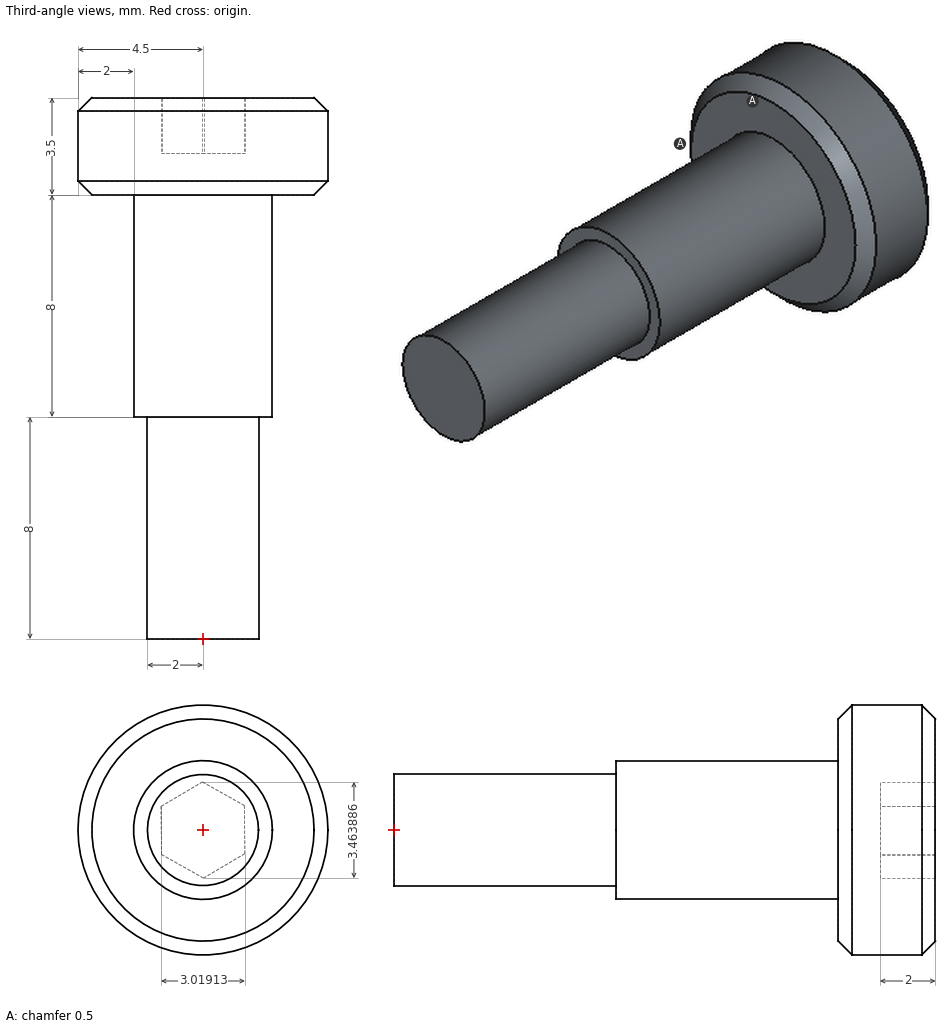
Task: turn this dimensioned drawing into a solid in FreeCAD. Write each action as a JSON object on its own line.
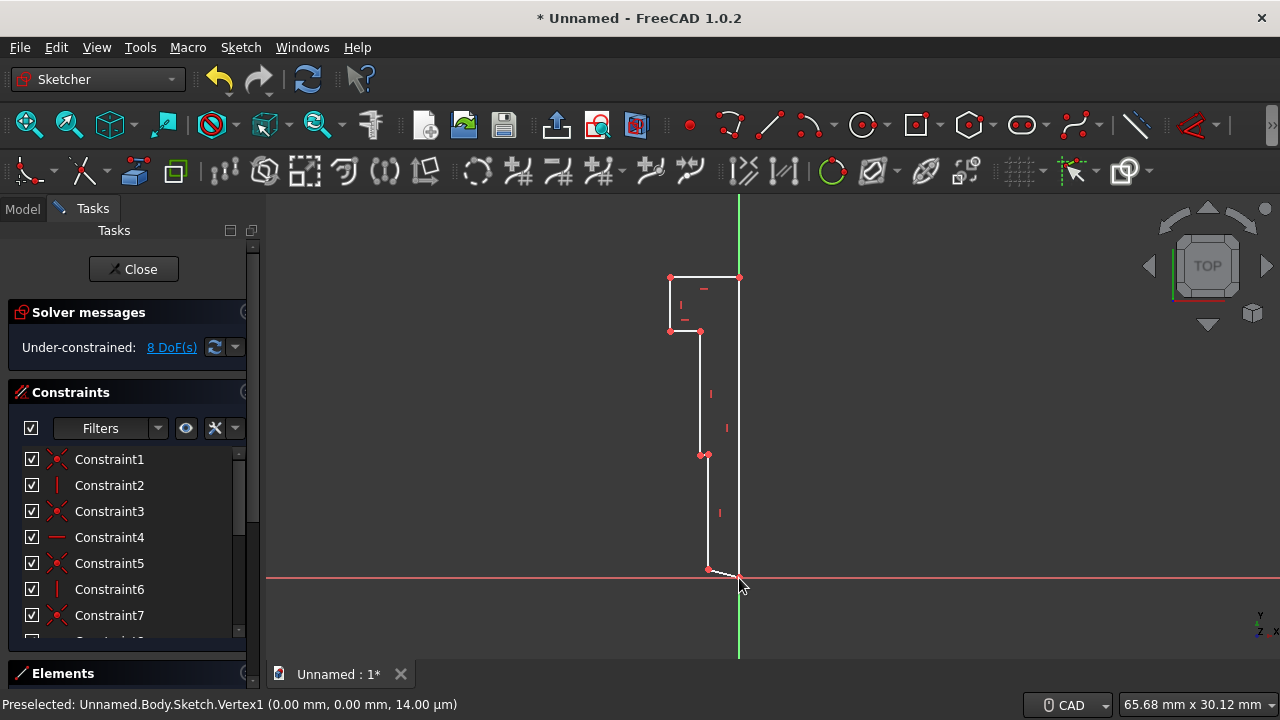
{"action": "scroll", "coordinate": [704, 455], "scroll_direction": "up", "scroll_amount": 7}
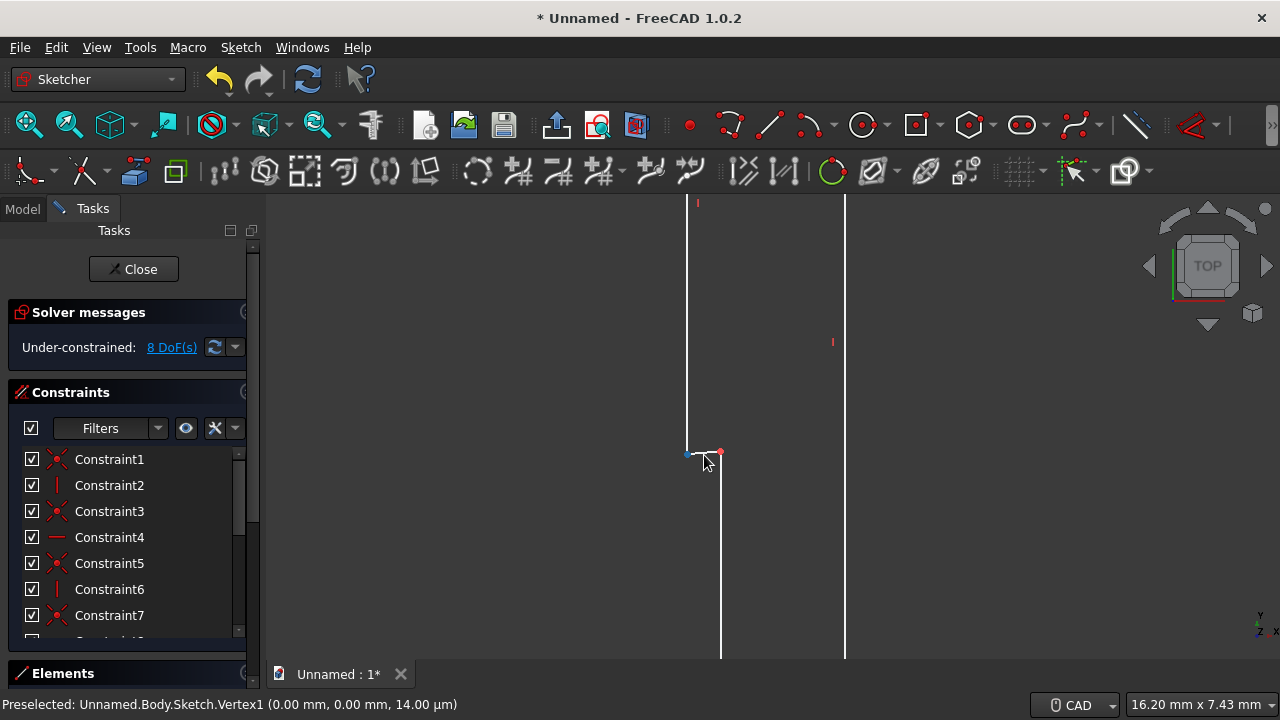
{"action": "left_click", "coordinate": [704, 453]}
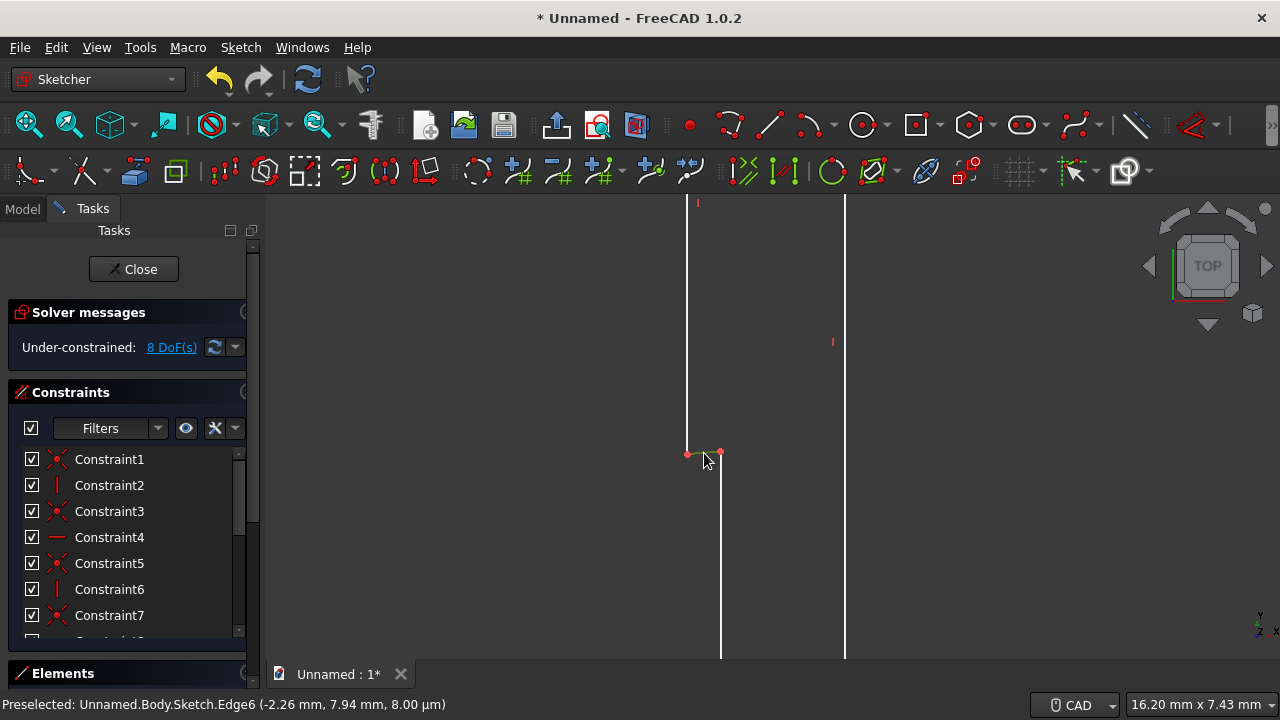
{"action": "key", "text": "h"}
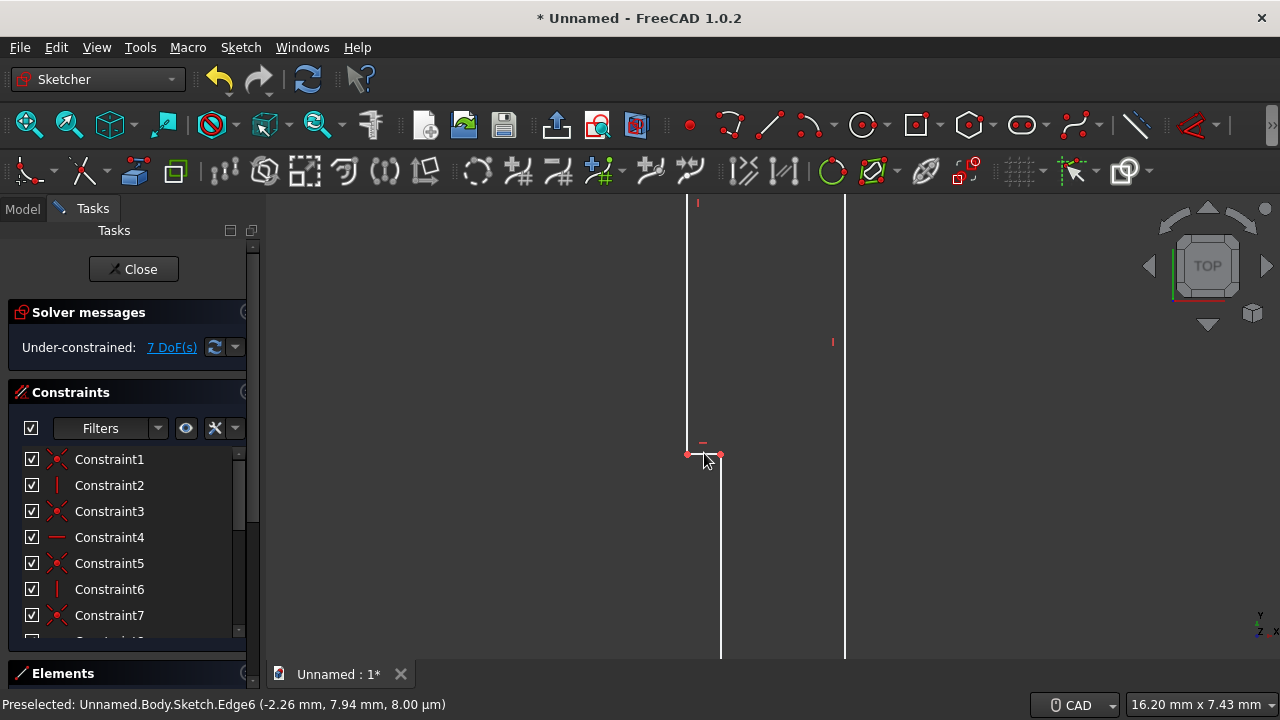
{"action": "scroll", "coordinate": [704, 455], "scroll_direction": "down", "scroll_amount": 7}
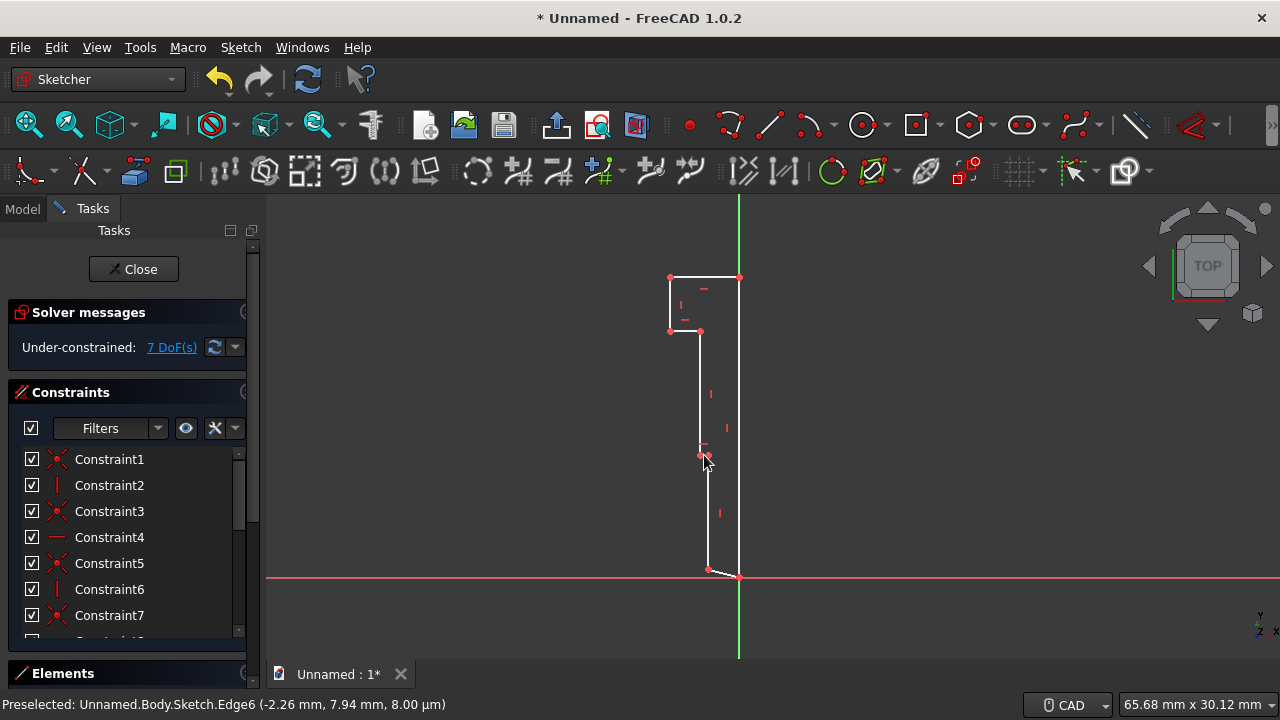
{"action": "scroll", "coordinate": [718, 572], "scroll_direction": "up", "scroll_amount": 5}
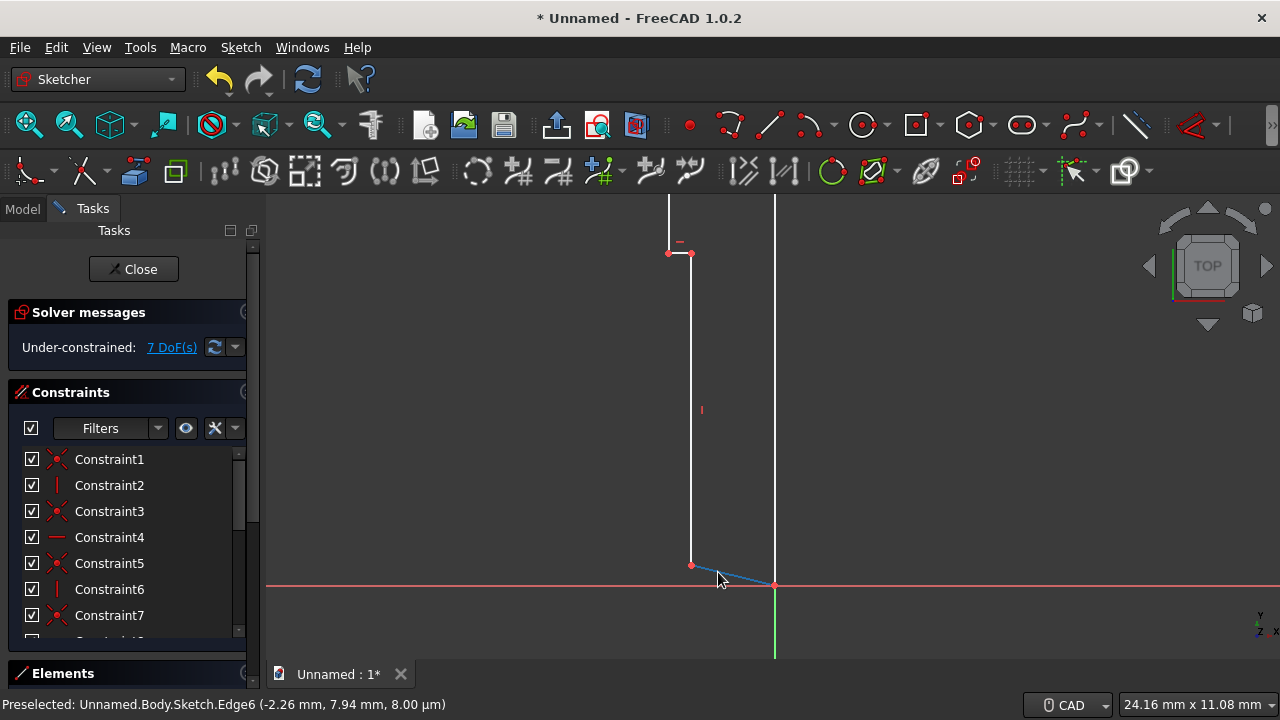
{"action": "left_click", "coordinate": [716, 571]}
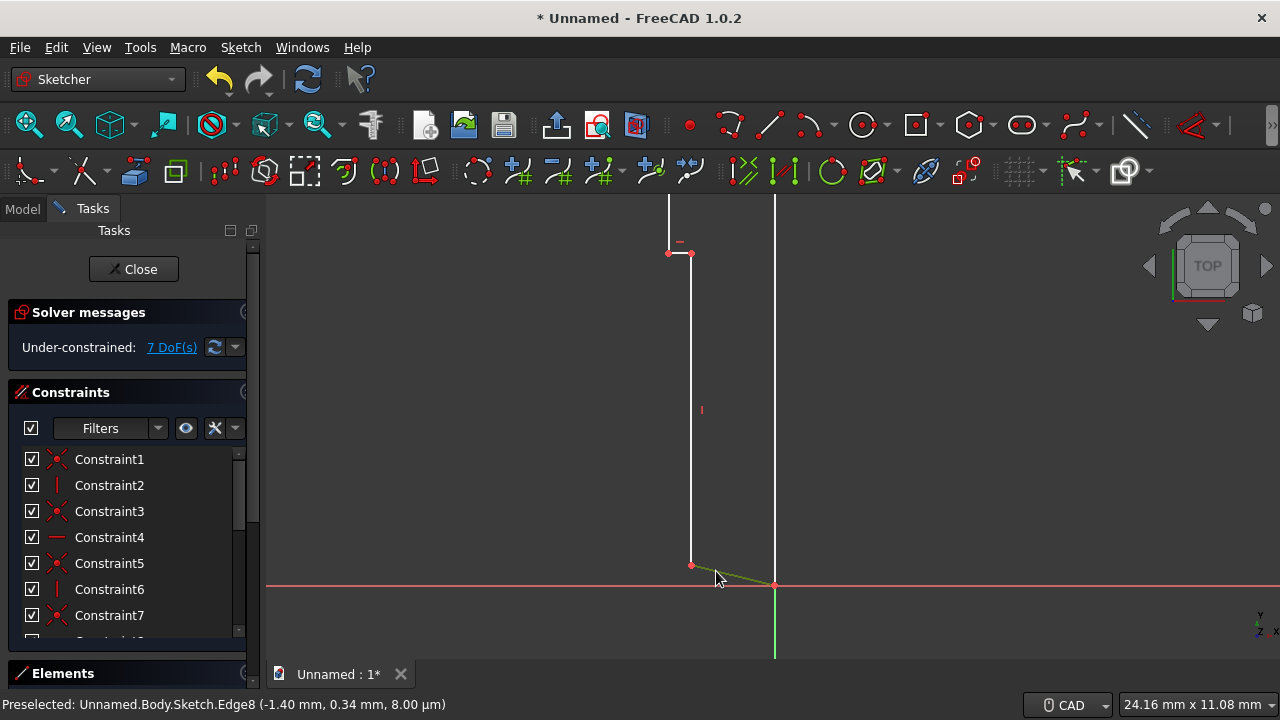
{"action": "key", "text": "h"}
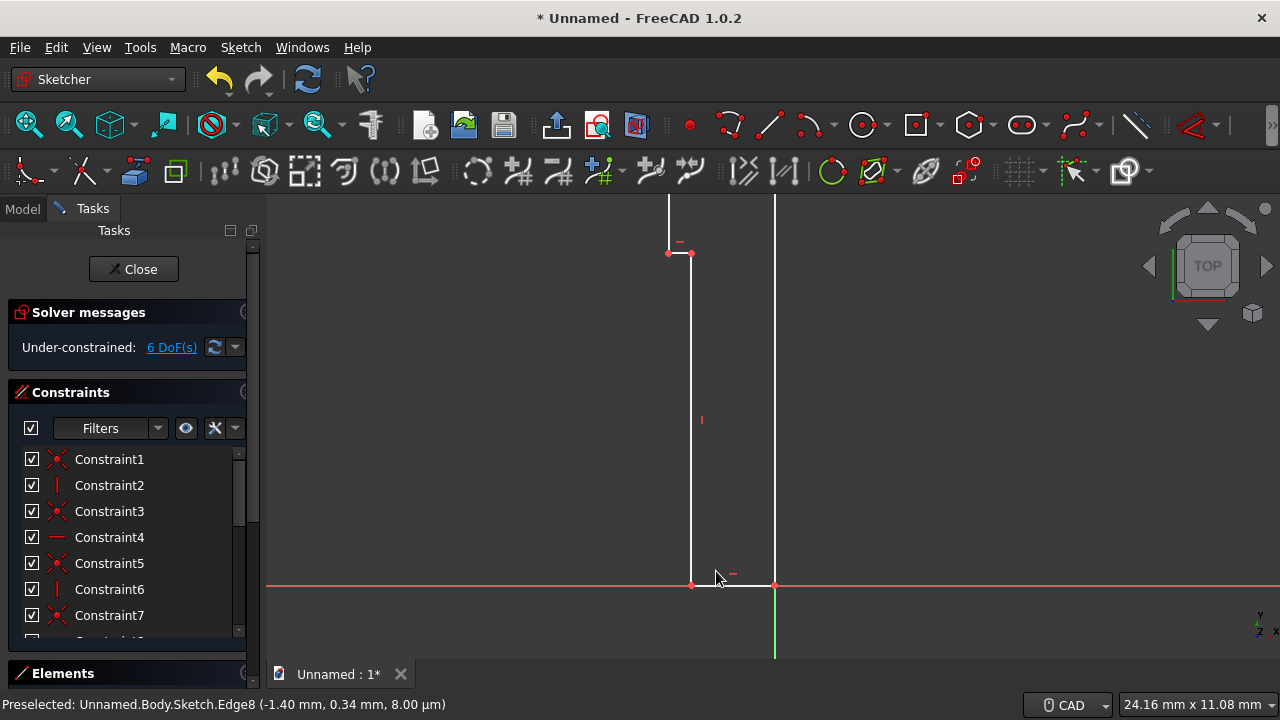
{"action": "left_click", "coordinate": [1192, 126]}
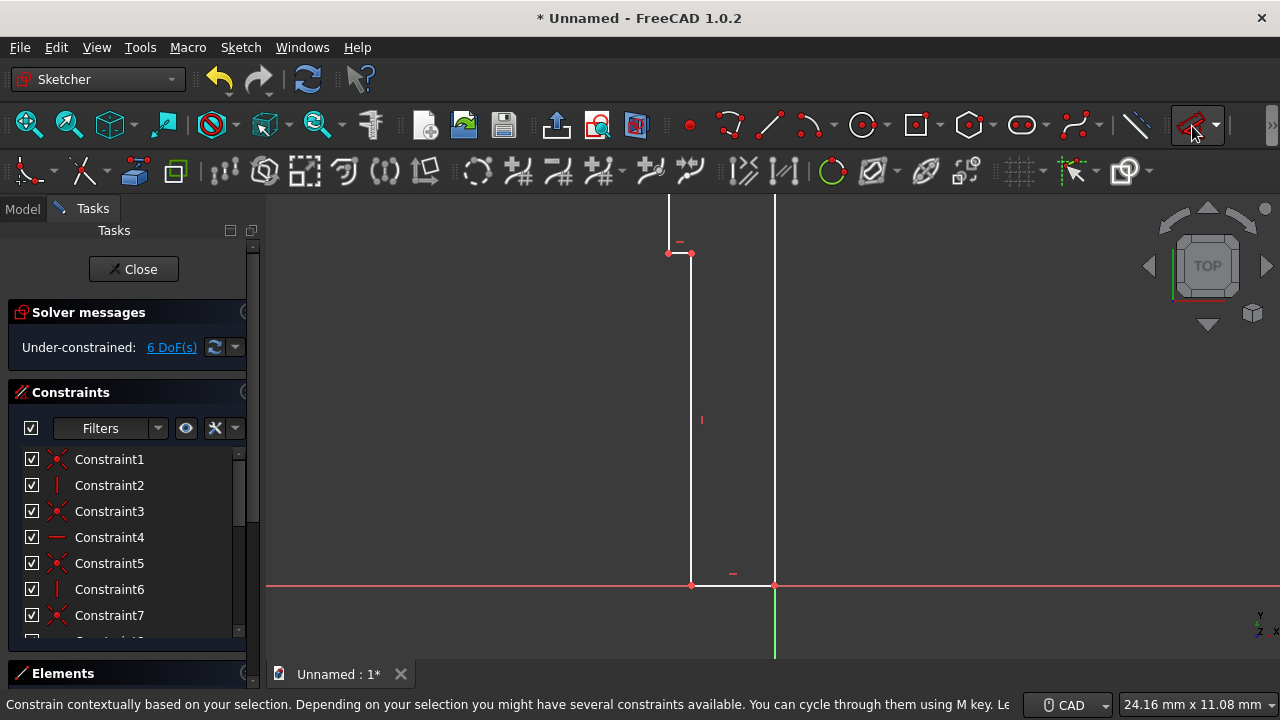
{"action": "scroll", "coordinate": [718, 572], "scroll_direction": "down", "scroll_amount": 5}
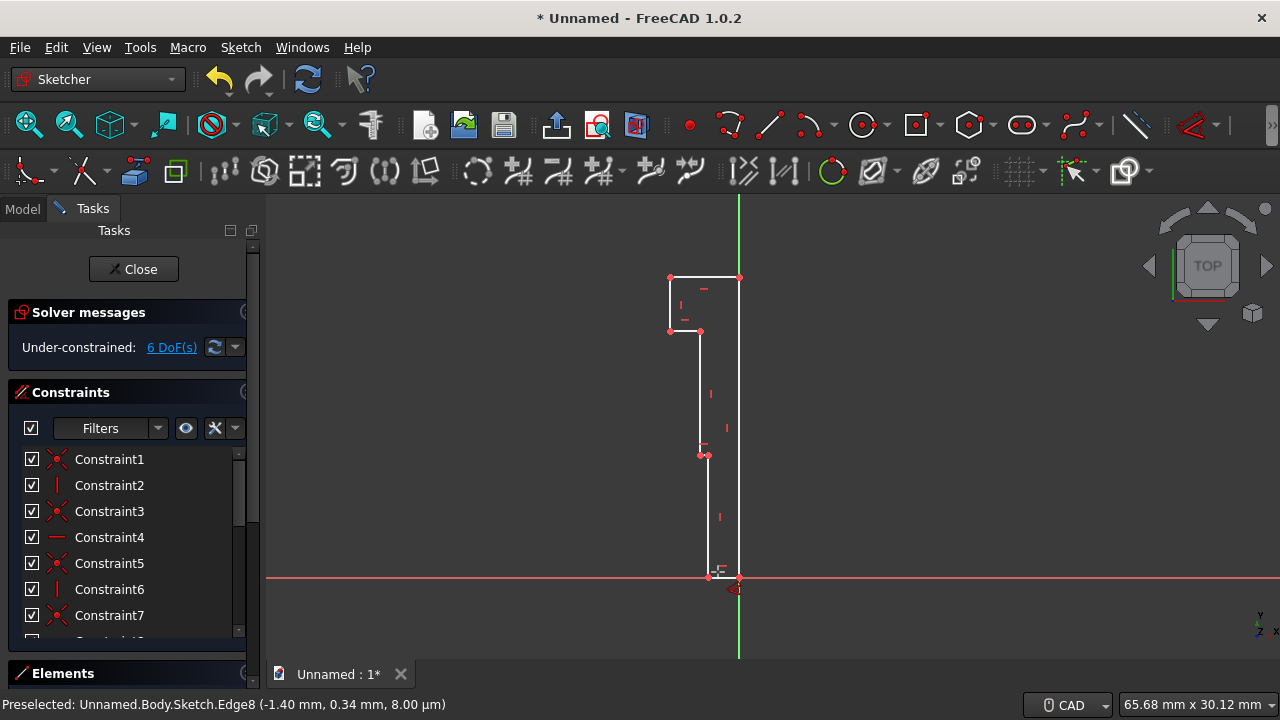
{"action": "scroll", "coordinate": [679, 331], "scroll_direction": "up", "scroll_amount": 3}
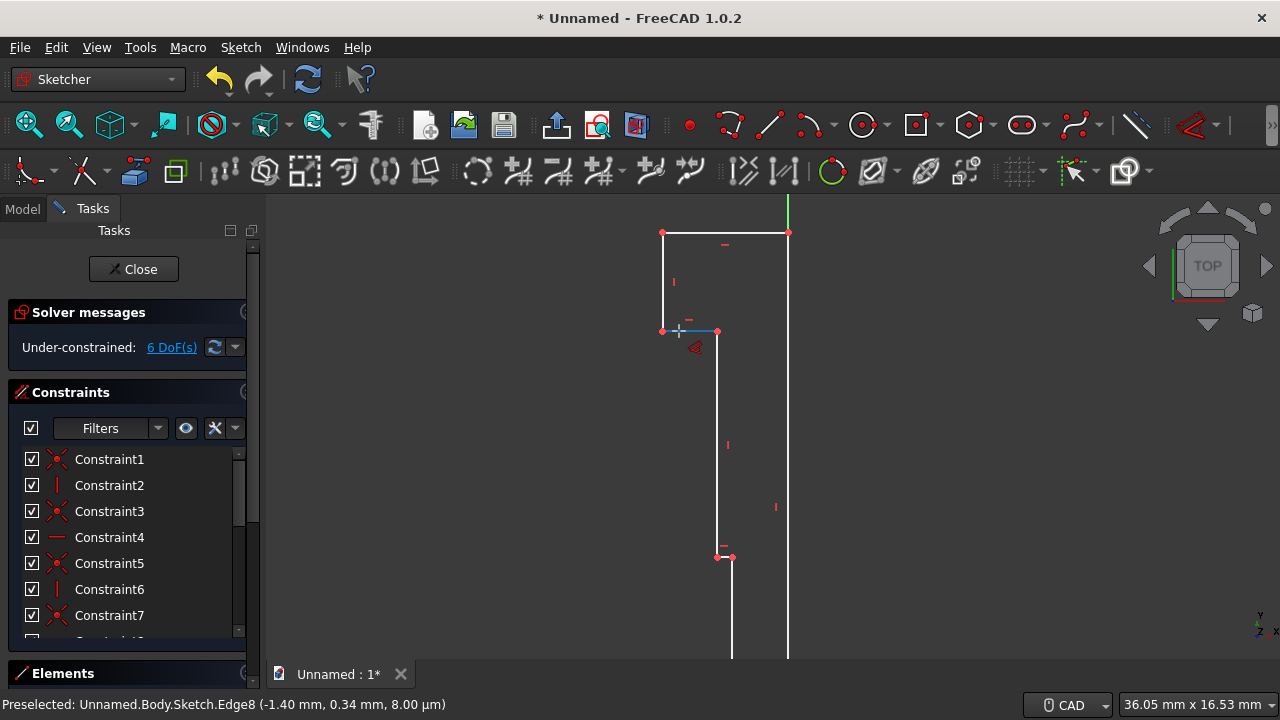
{"action": "left_click", "coordinate": [679, 331]}
{"action": "left_click", "coordinate": [690, 297]}